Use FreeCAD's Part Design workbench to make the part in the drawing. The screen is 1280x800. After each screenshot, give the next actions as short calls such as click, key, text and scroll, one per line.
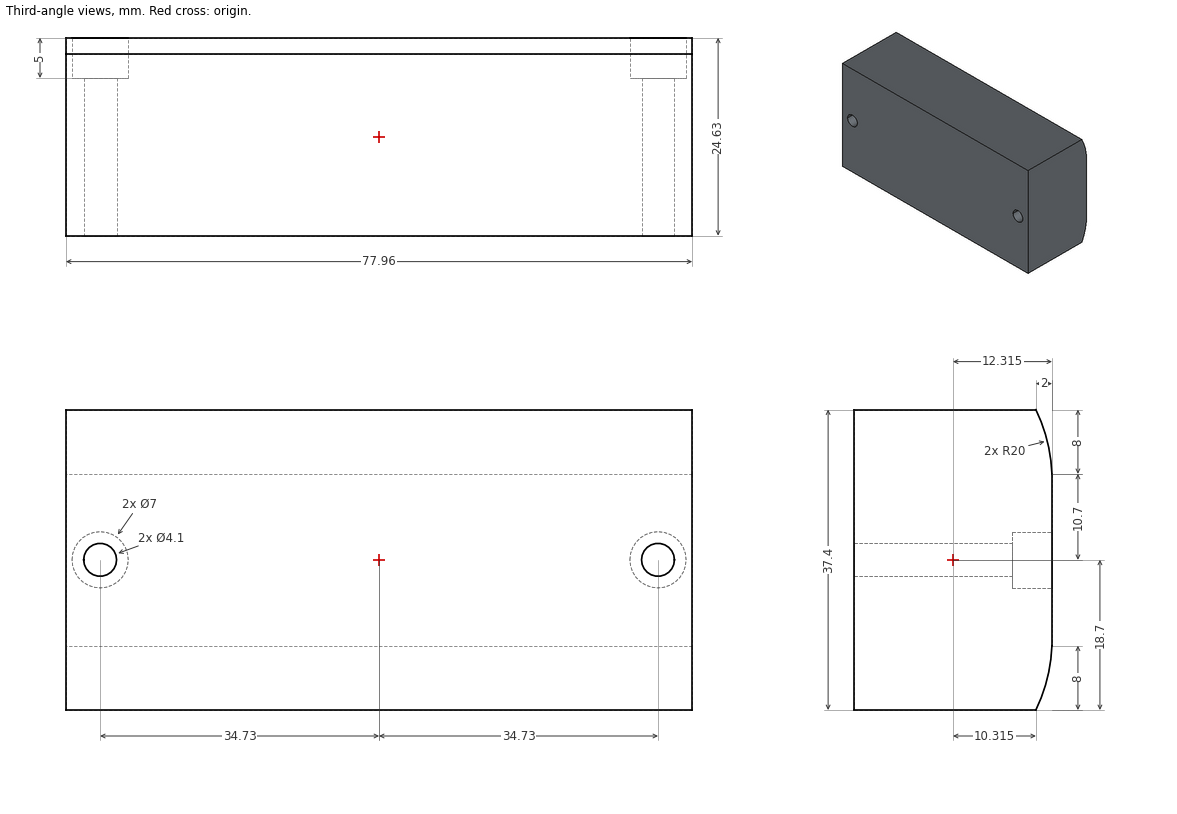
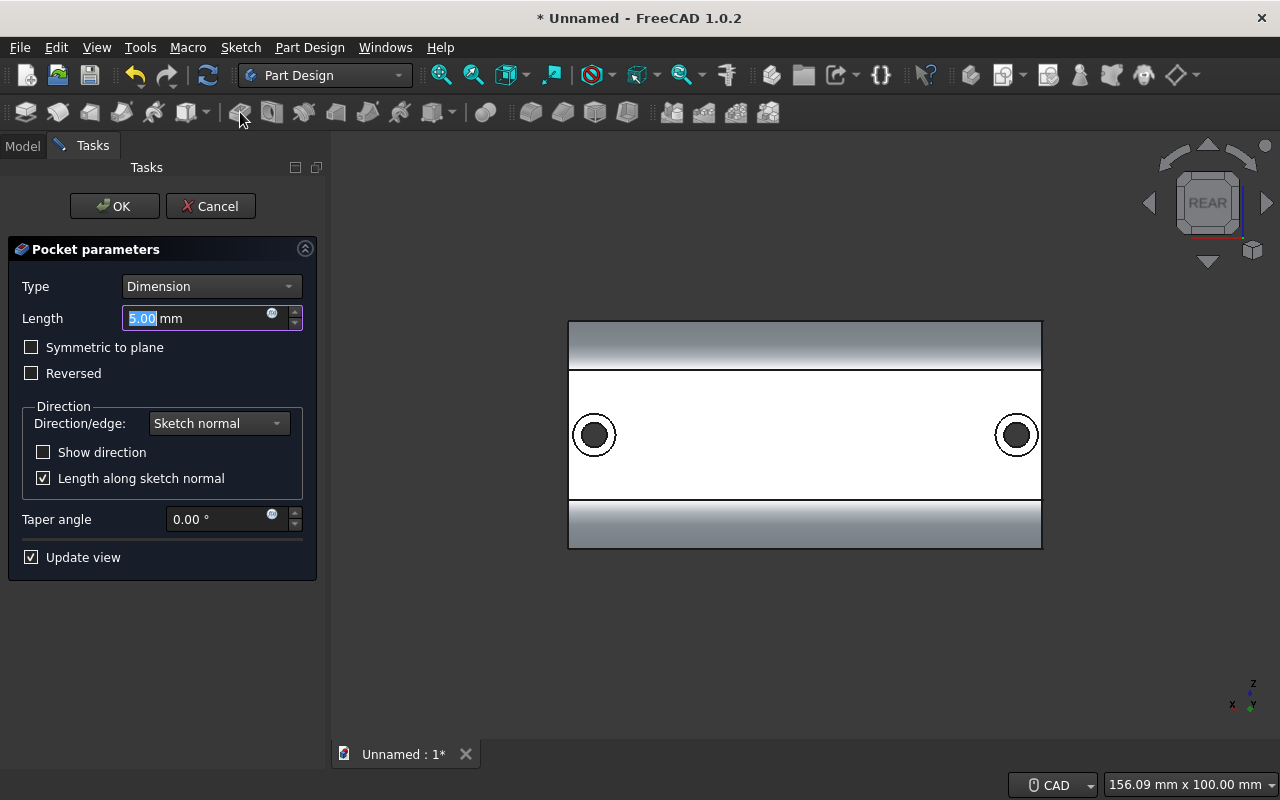
text(5)
key(Tab)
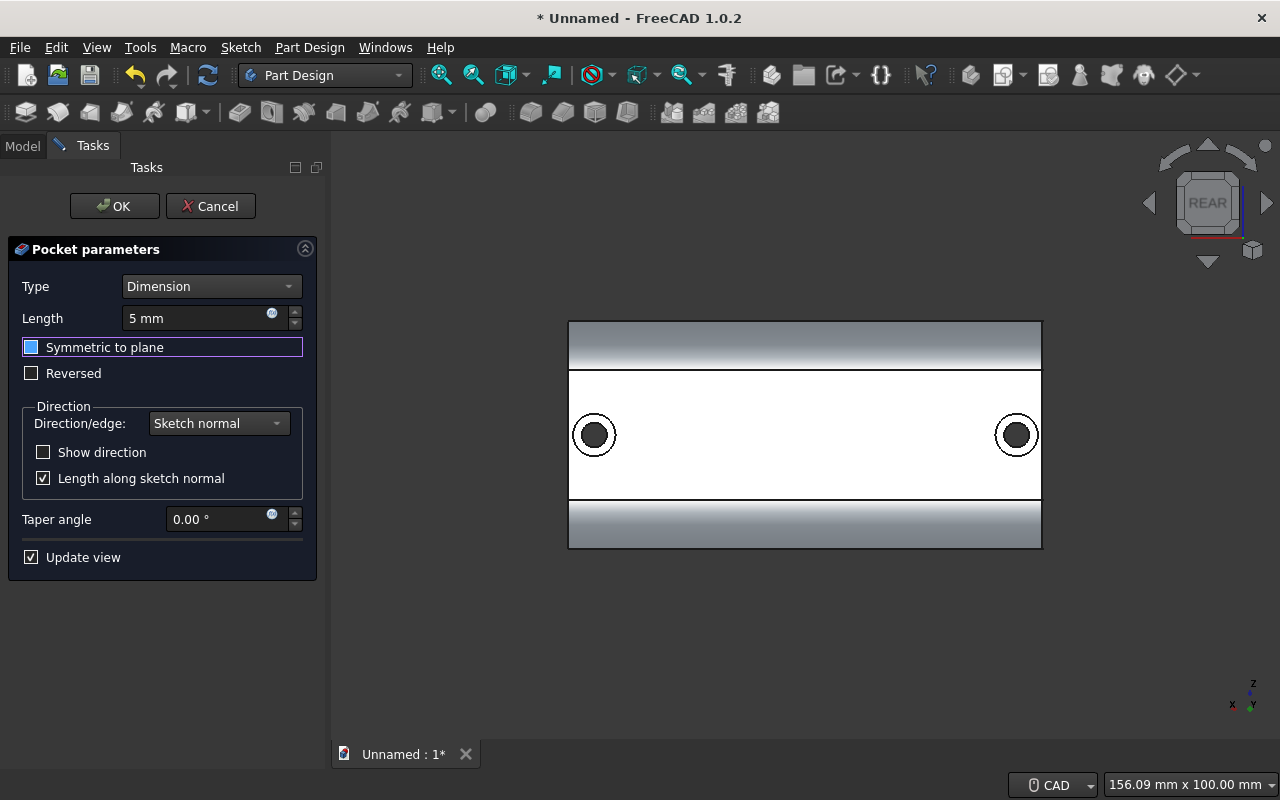
click(115, 206)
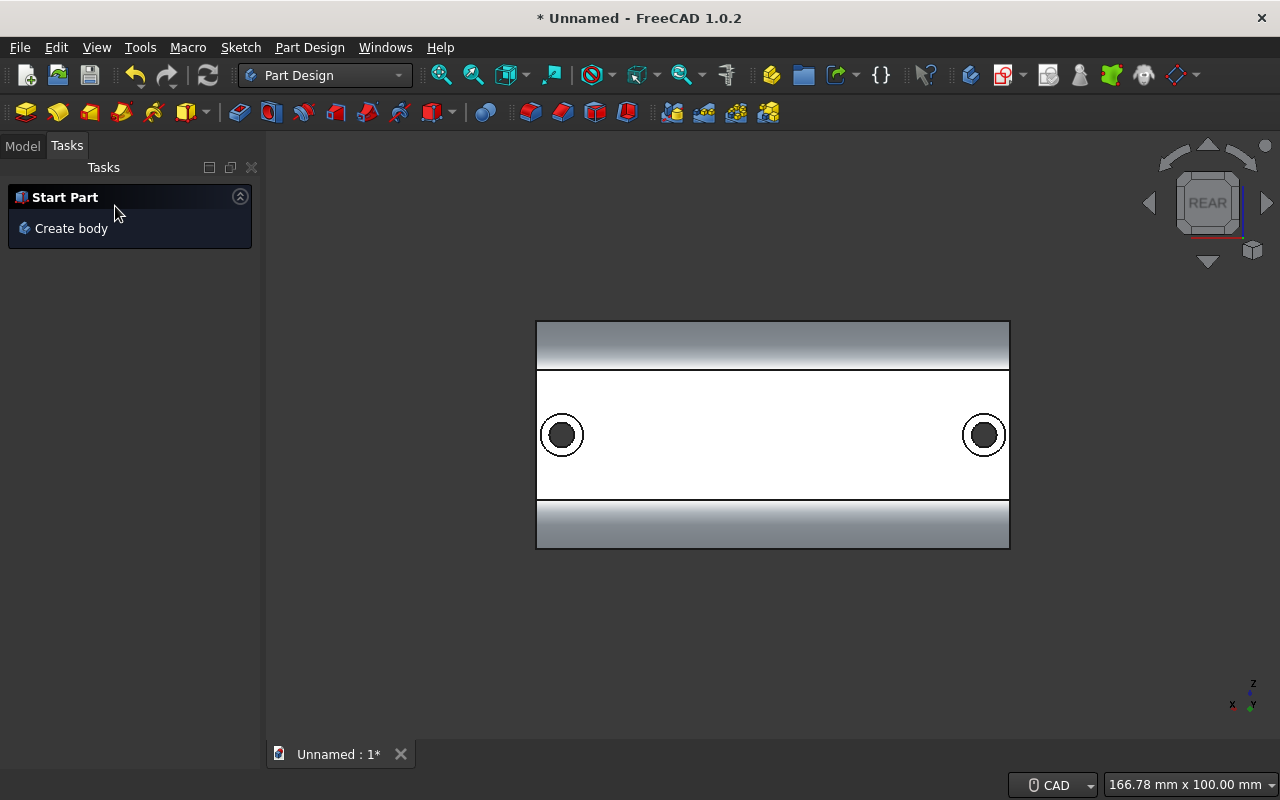
key(0)